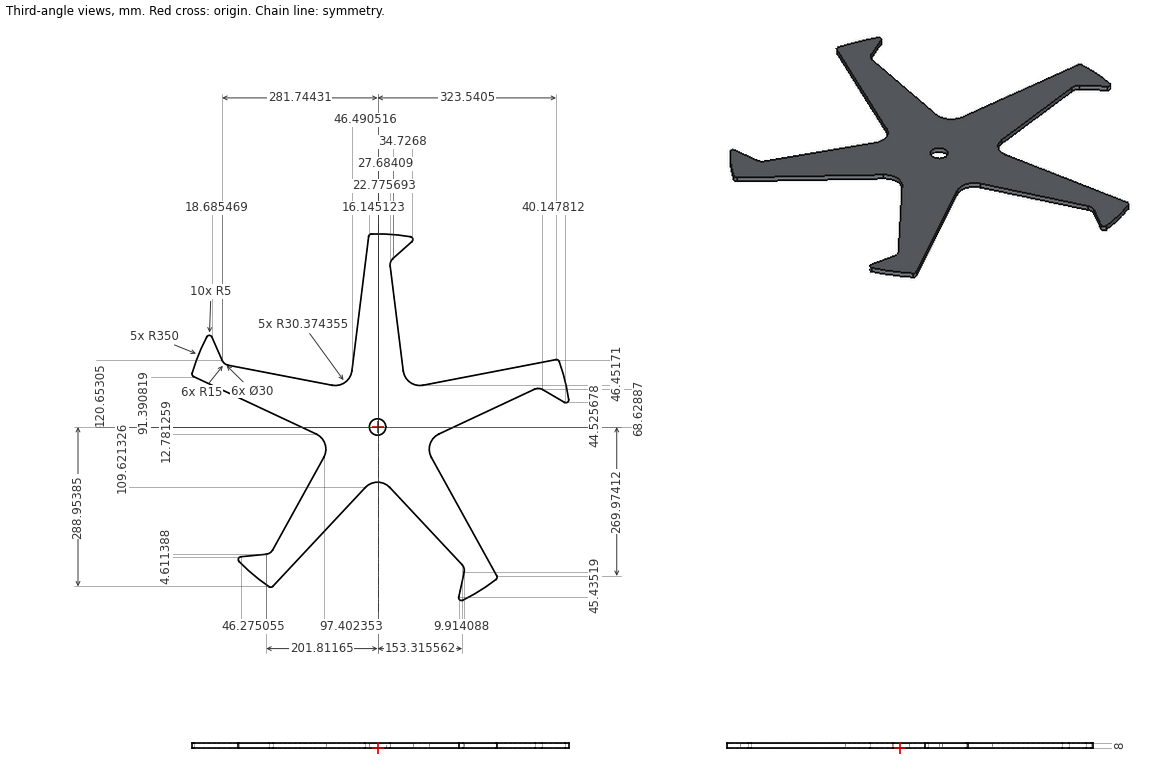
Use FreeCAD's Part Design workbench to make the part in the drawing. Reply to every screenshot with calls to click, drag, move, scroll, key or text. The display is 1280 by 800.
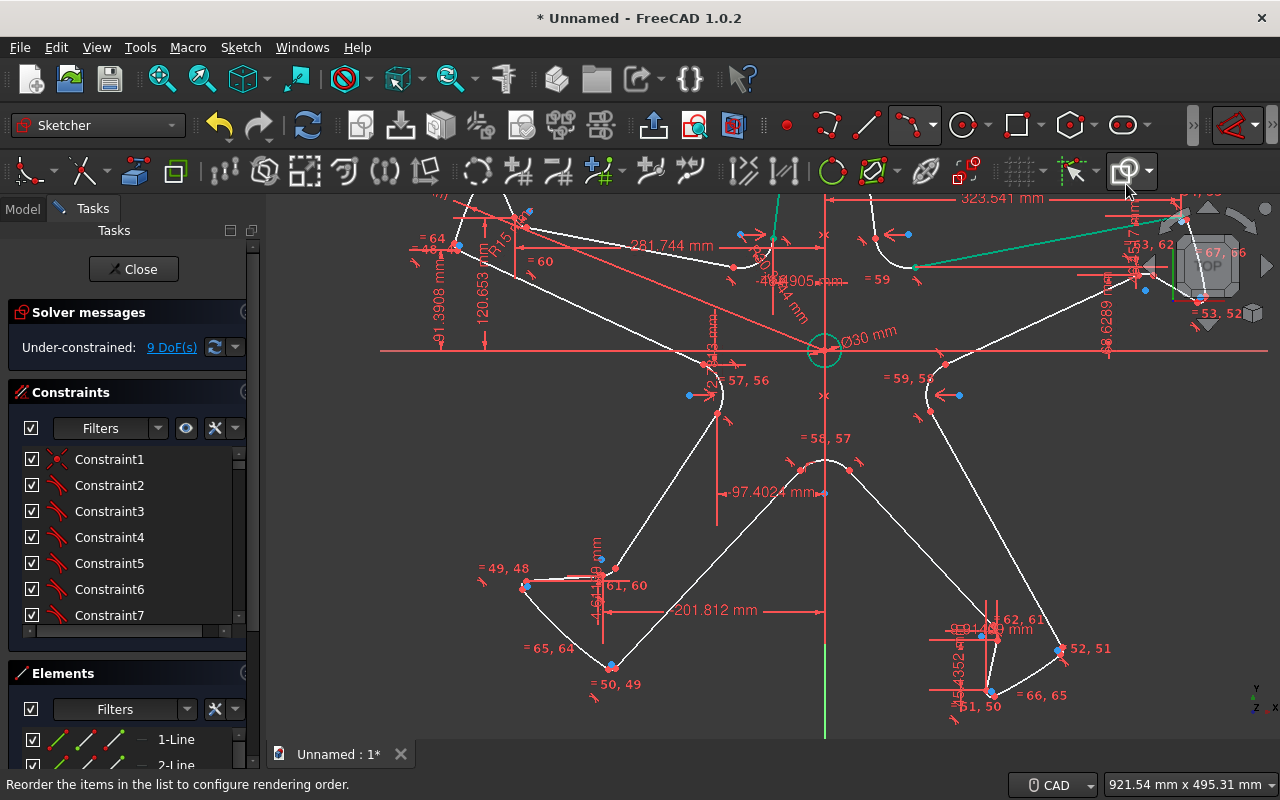
scroll(615, 668, up, 4)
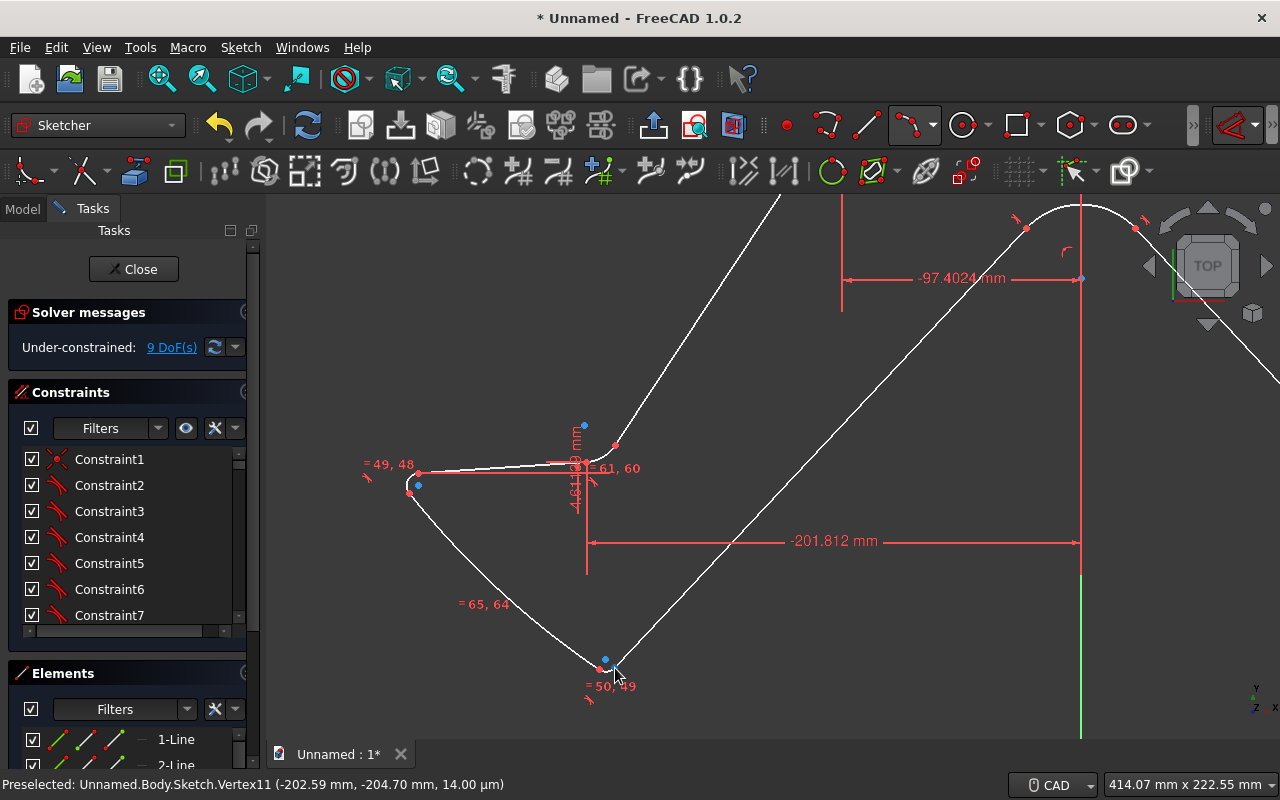
click(615, 668)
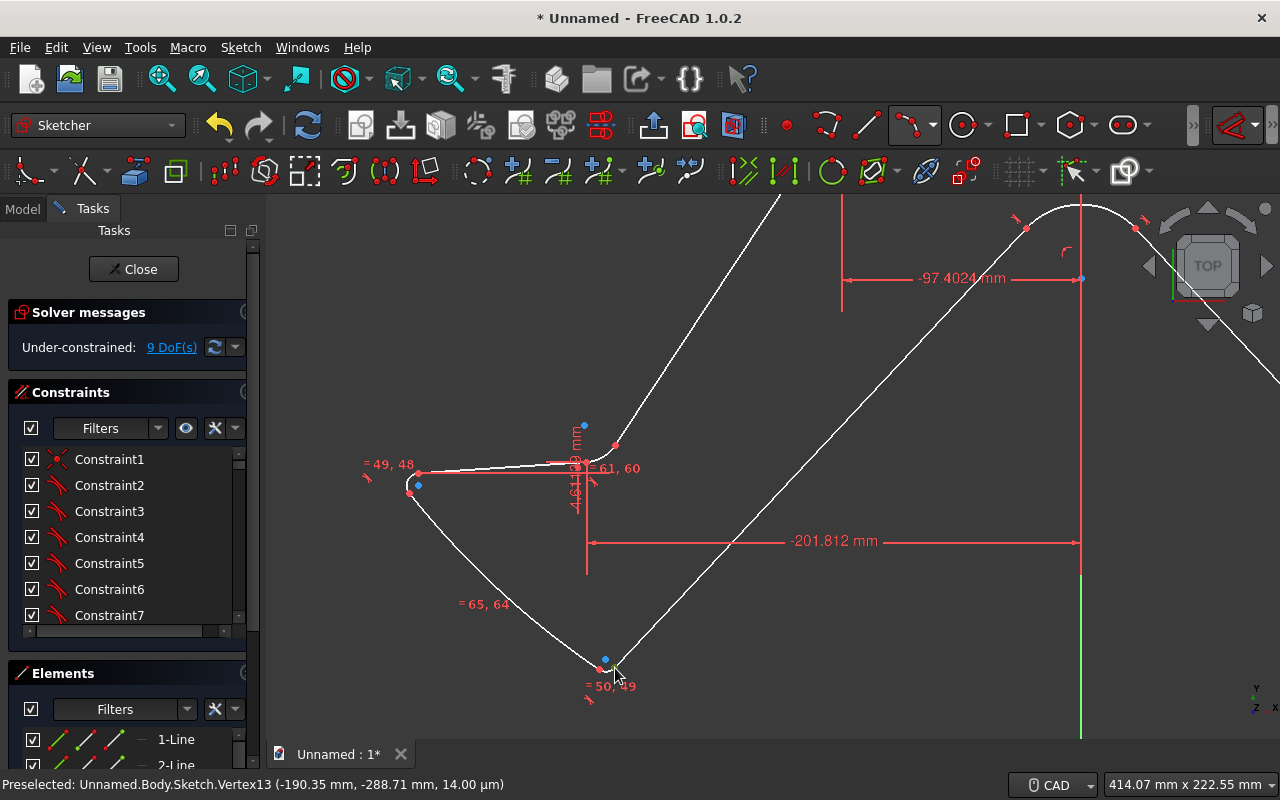
click(1258, 126)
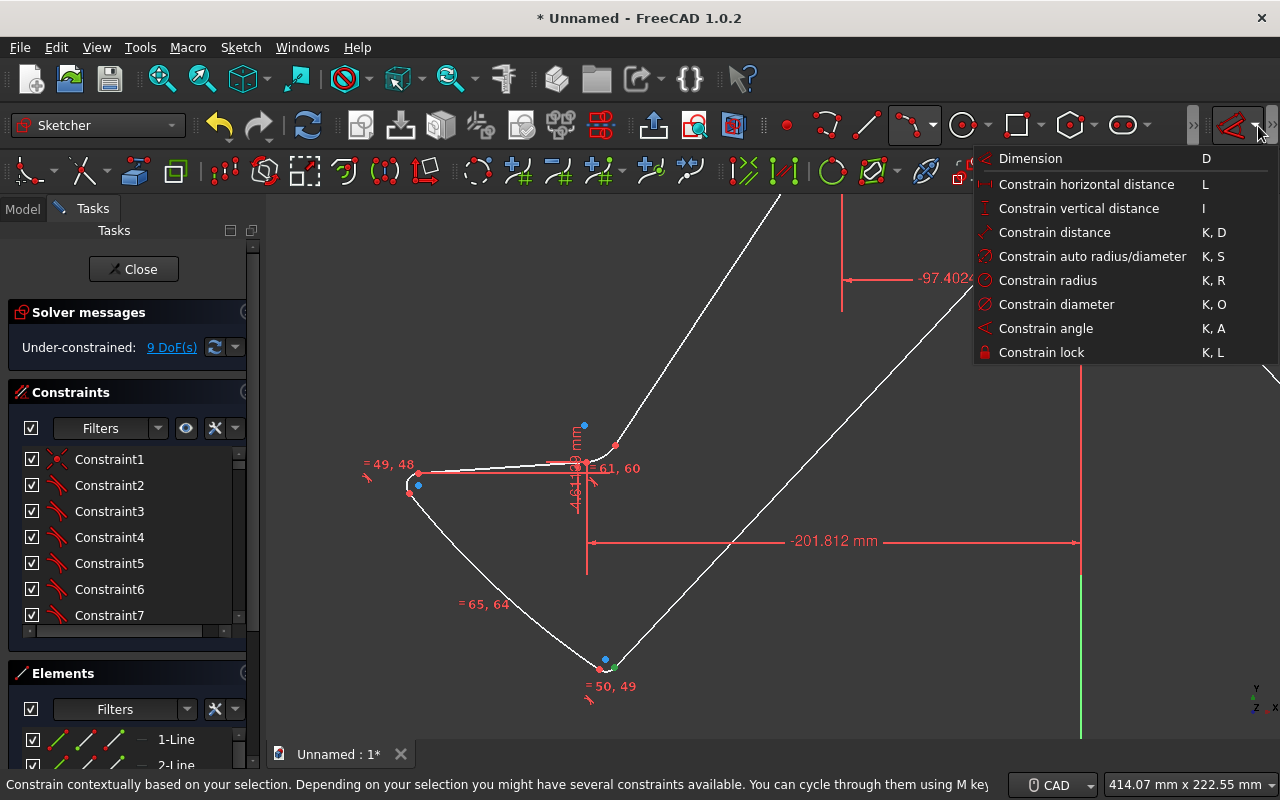
click(1126, 208)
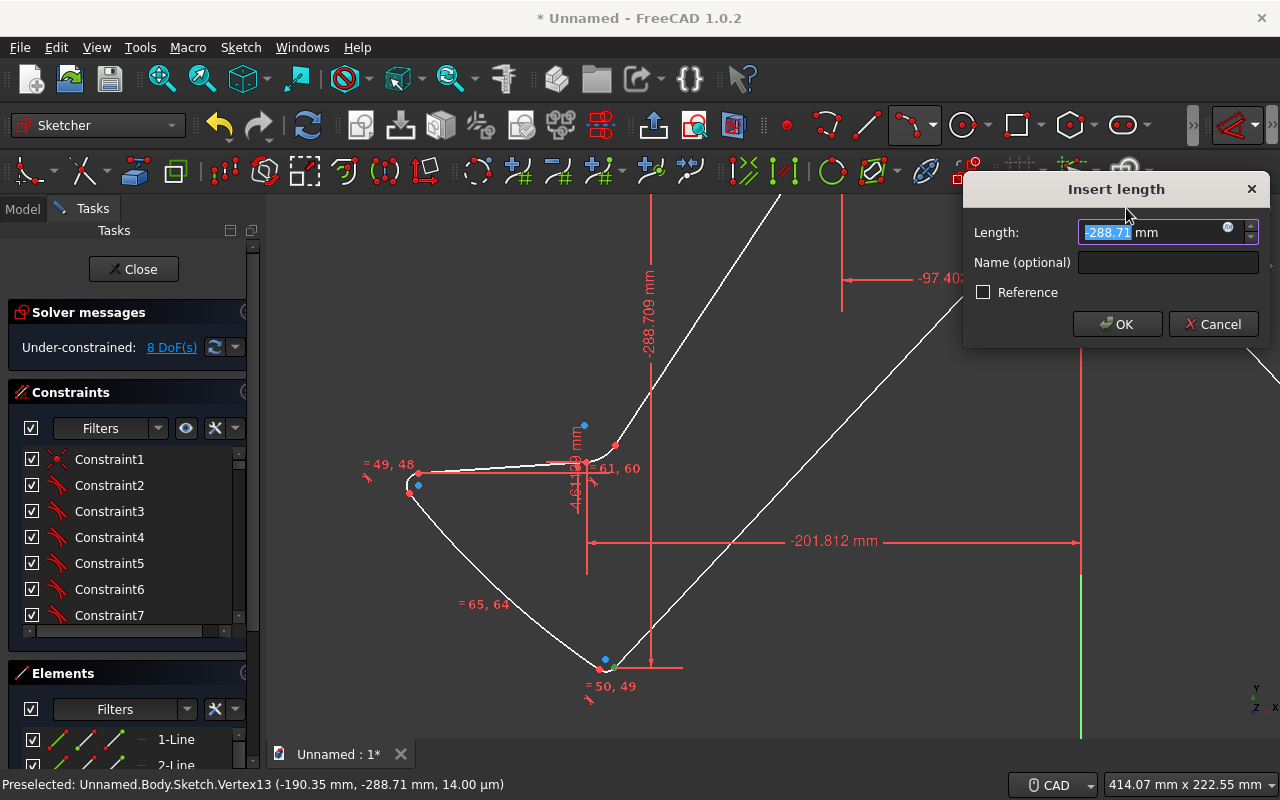
text(-288.95385)
key(Return)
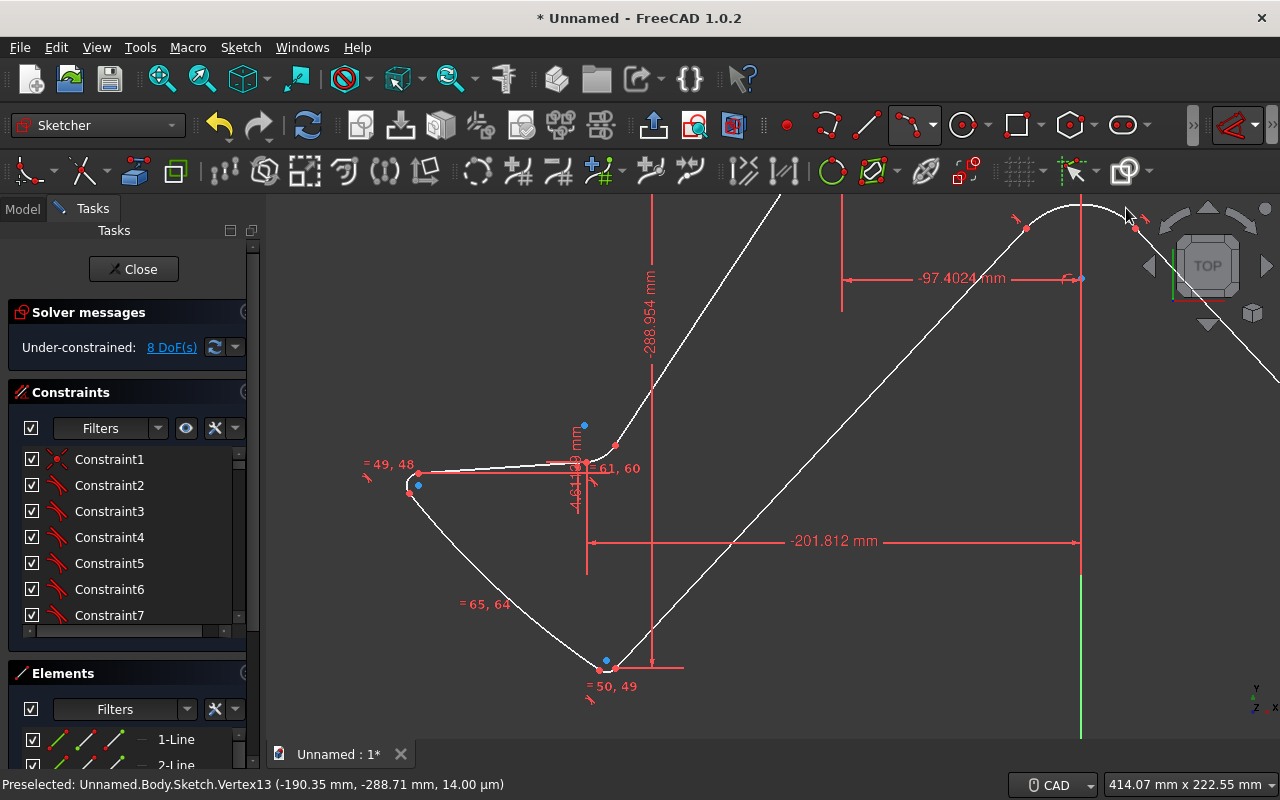
scroll(606, 605, down, 8)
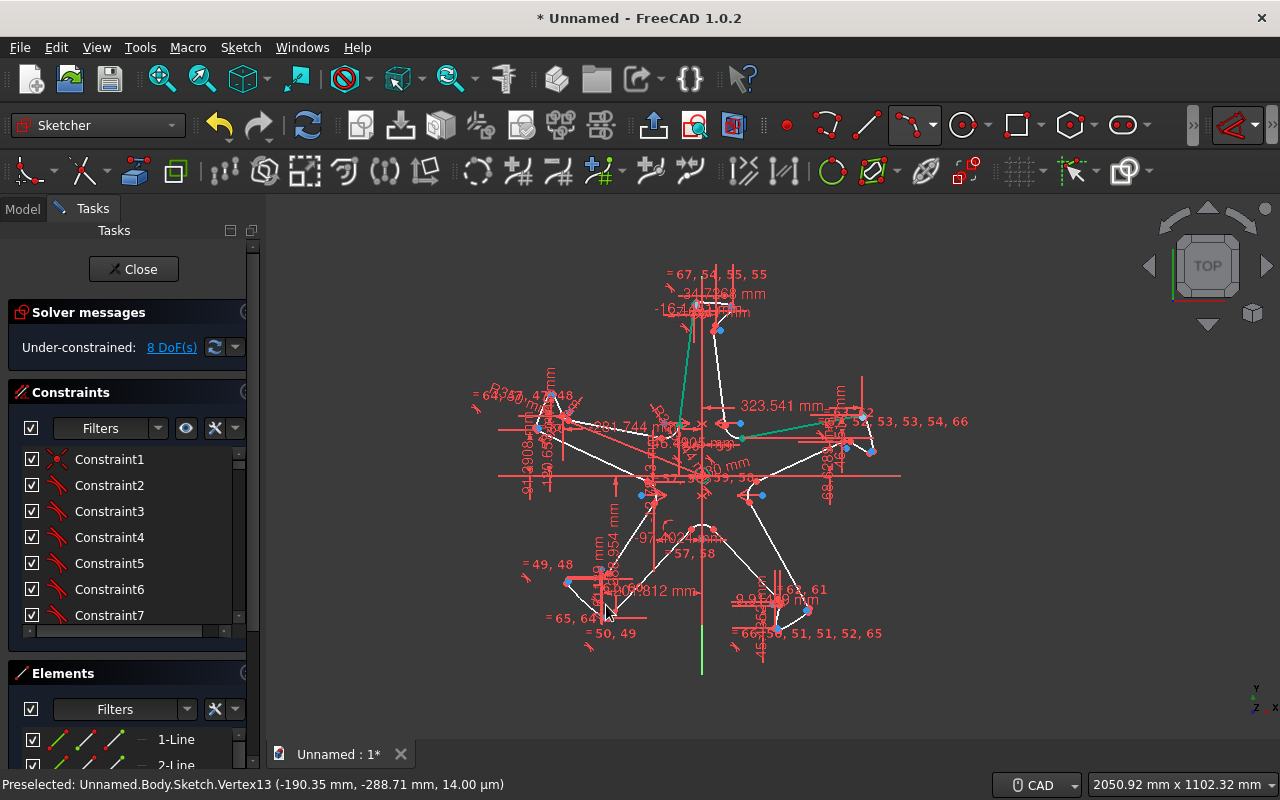
scroll(809, 609, up, 8)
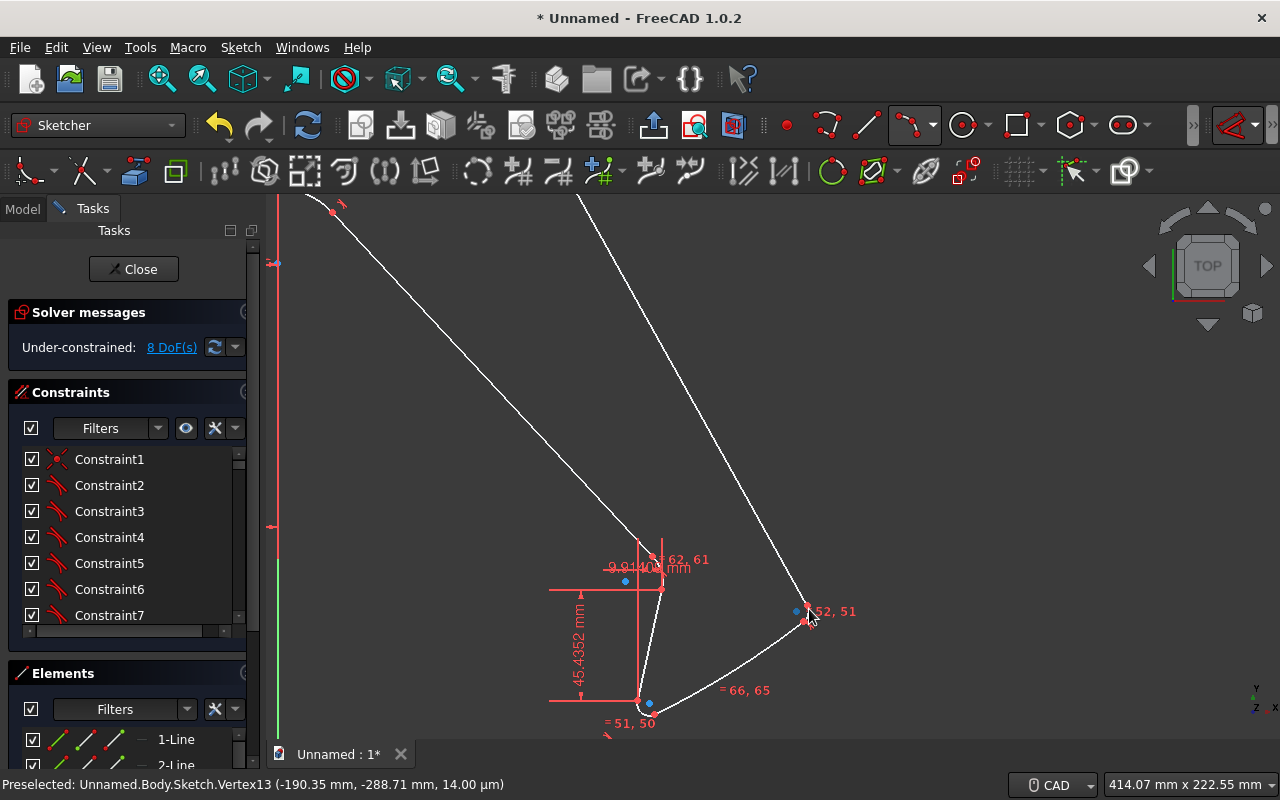
click(807, 606)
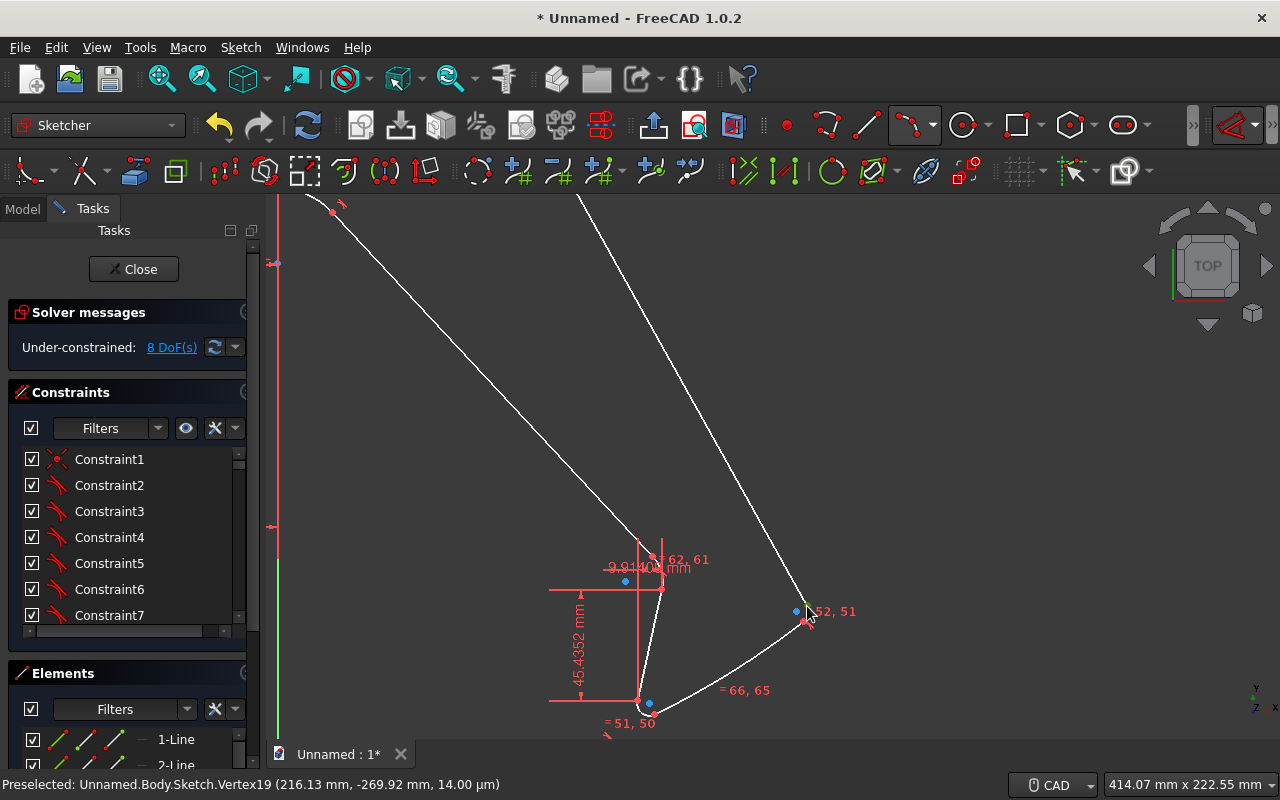
click(1258, 126)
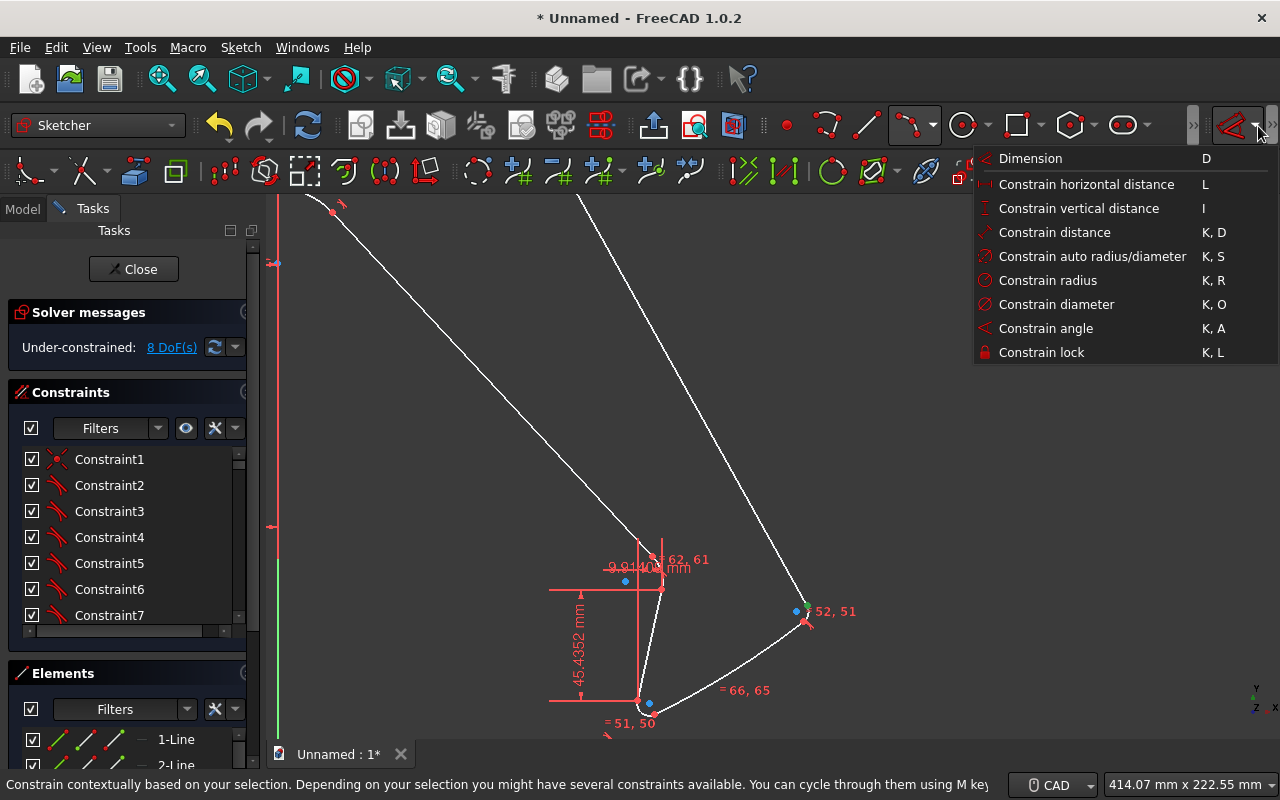
click(1126, 208)